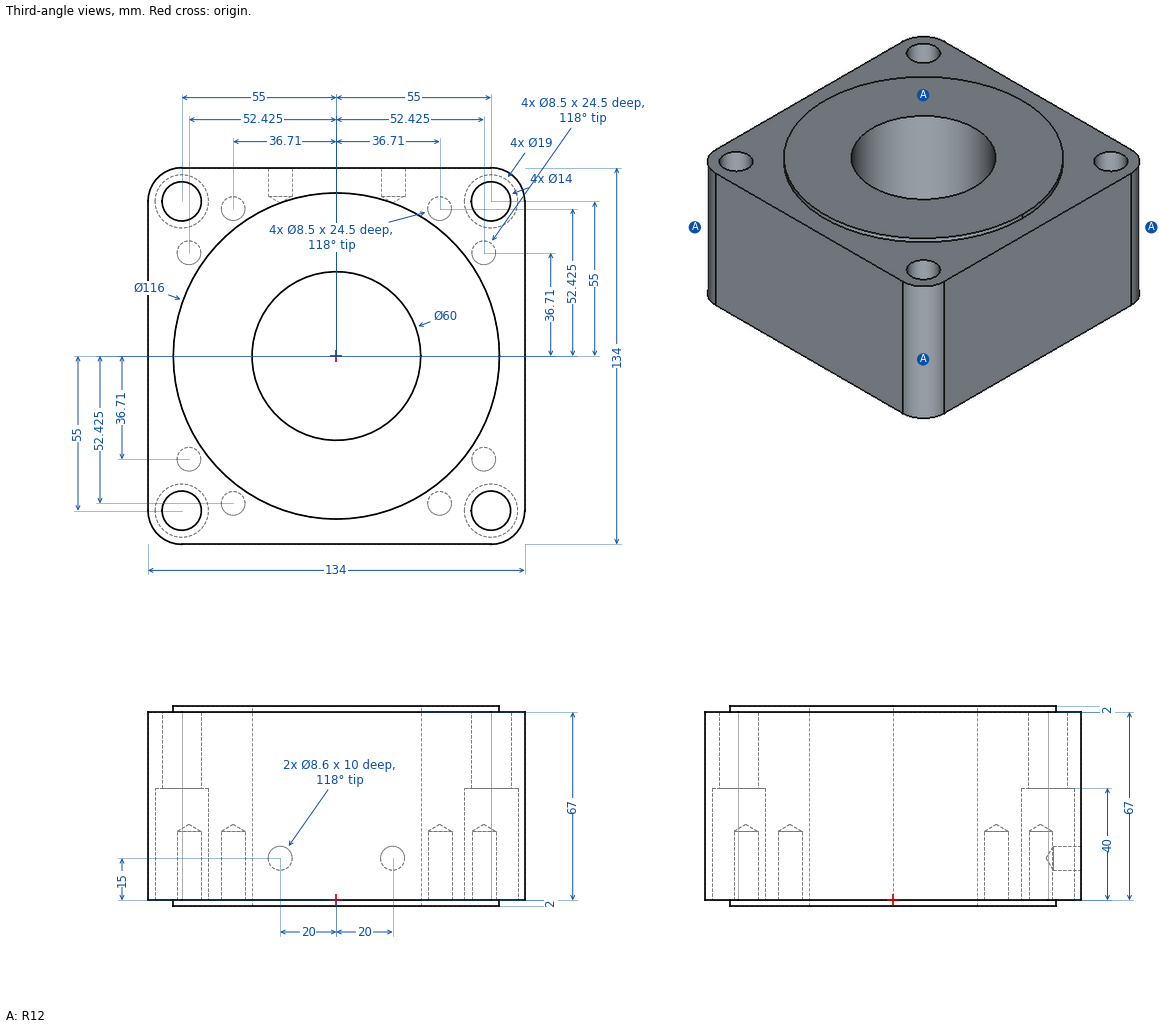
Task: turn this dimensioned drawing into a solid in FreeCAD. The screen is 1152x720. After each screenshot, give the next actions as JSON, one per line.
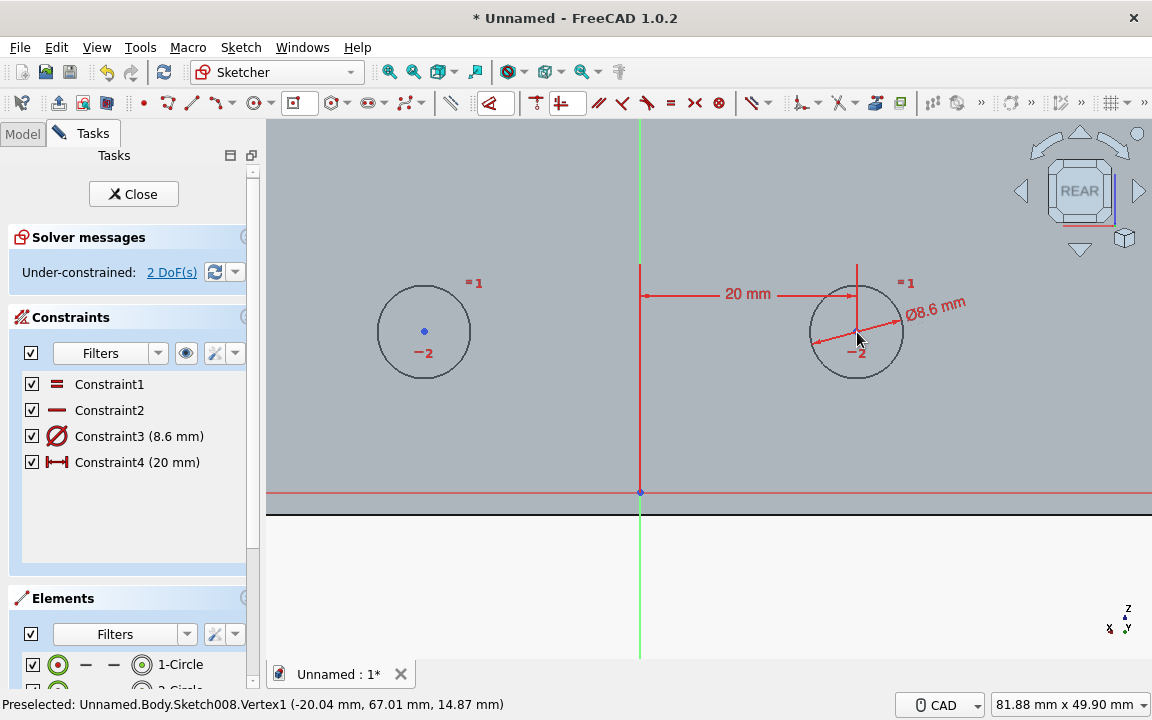
{"action": "left_click", "coordinate": [857, 332]}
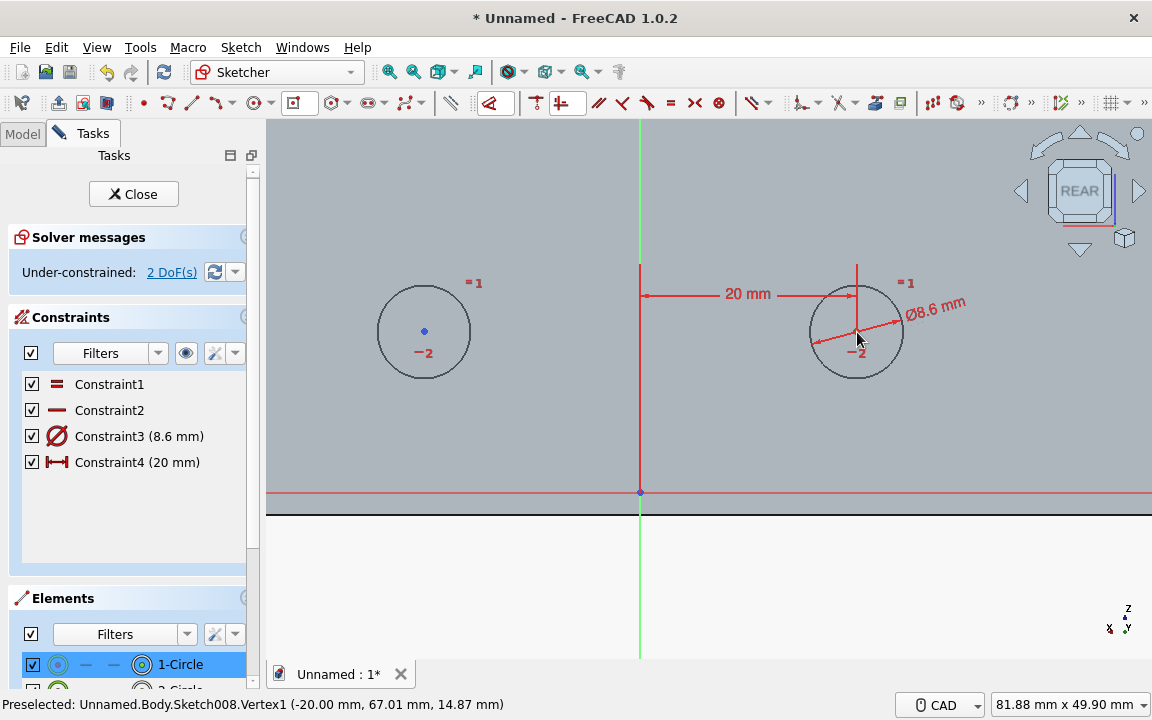
{"action": "key", "text": "i"}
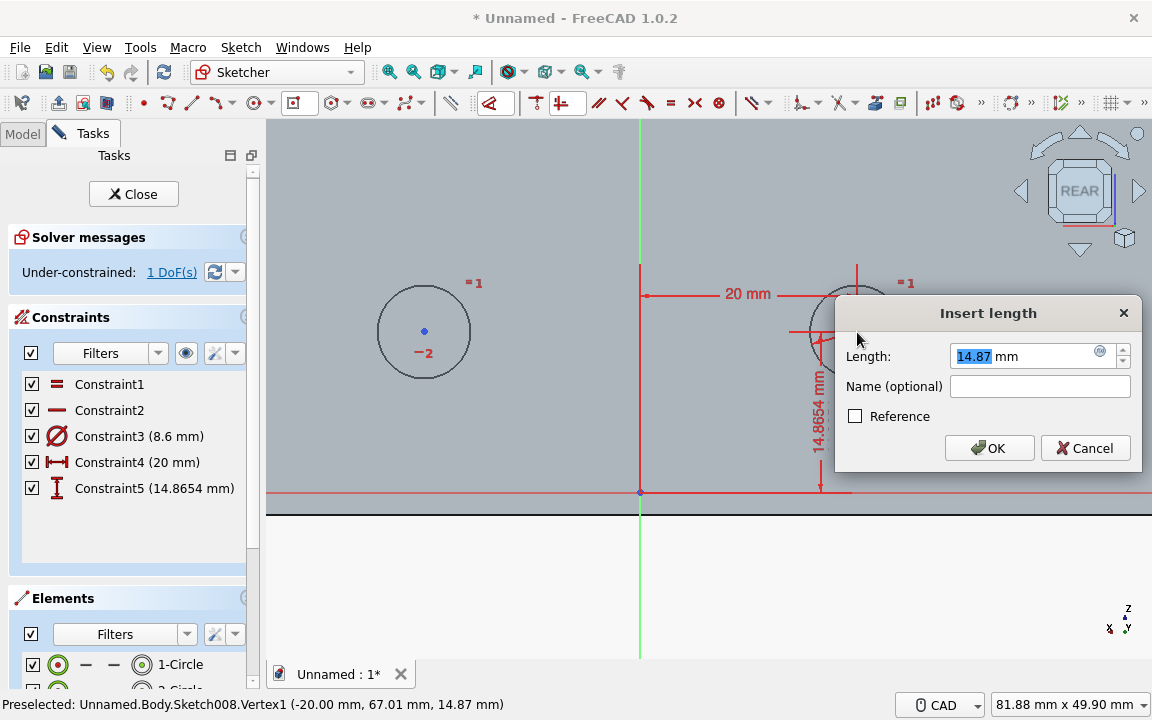
{"action": "type", "text": "15"}
{"action": "key", "text": "Return"}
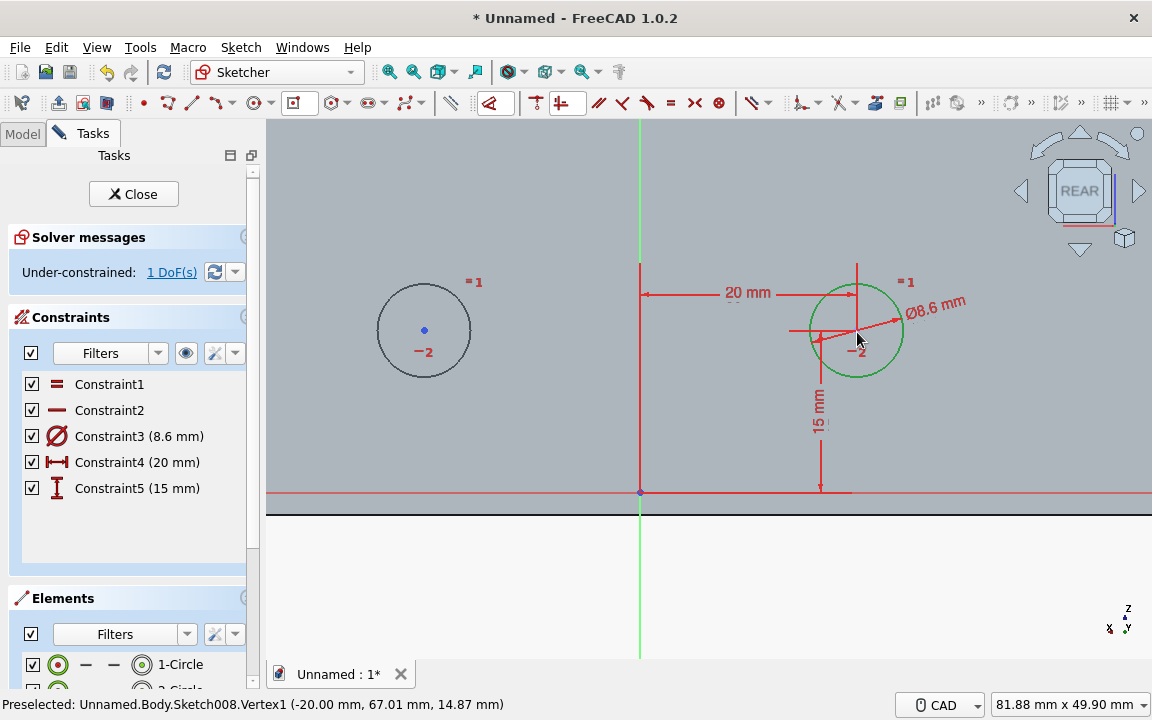
{"action": "left_click", "coordinate": [424, 331]}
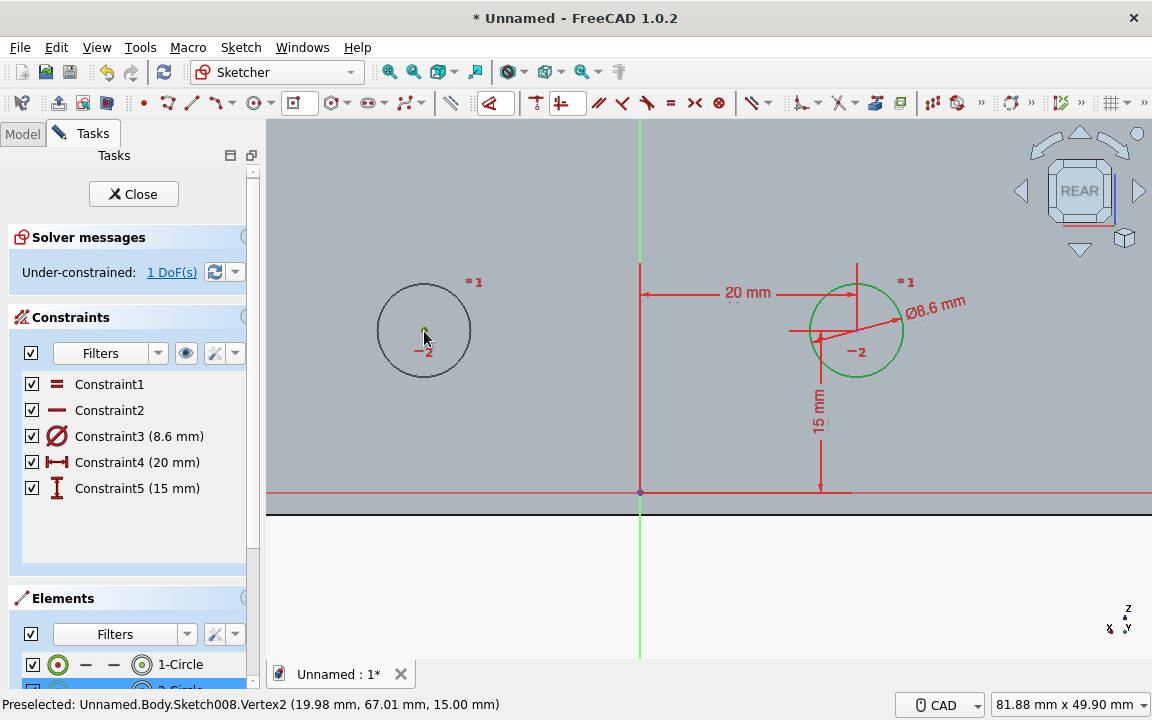
{"action": "left_click", "coordinate": [508, 104]}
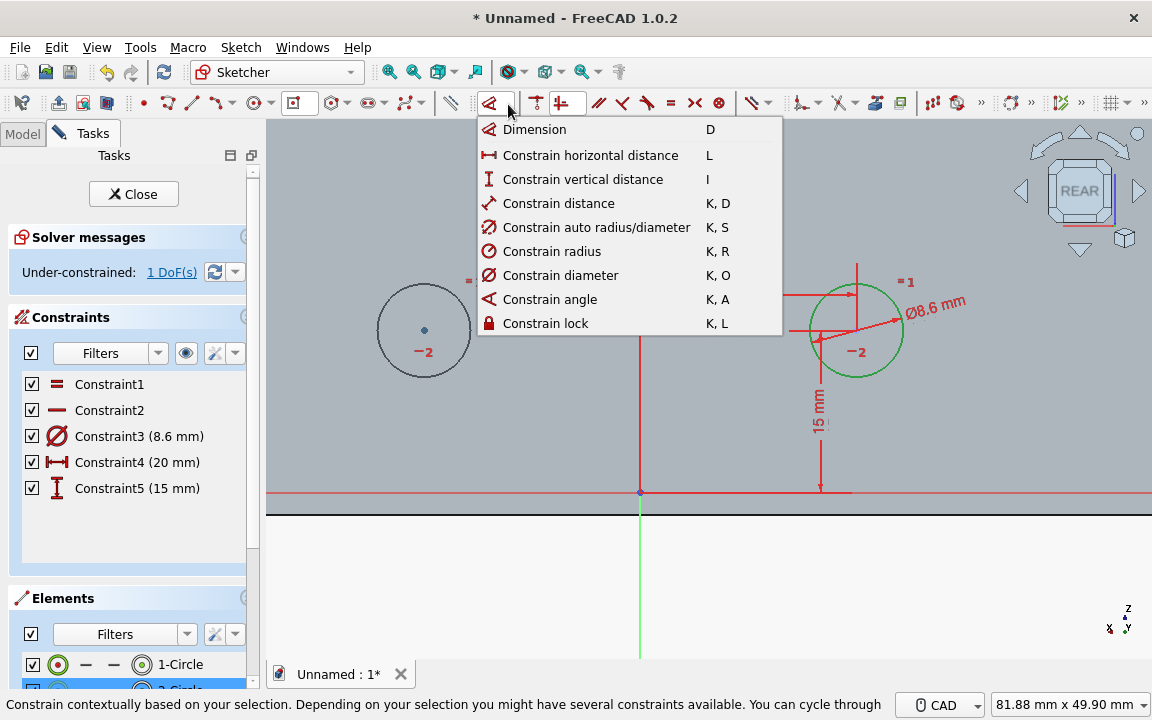
{"action": "left_click", "coordinate": [630, 155]}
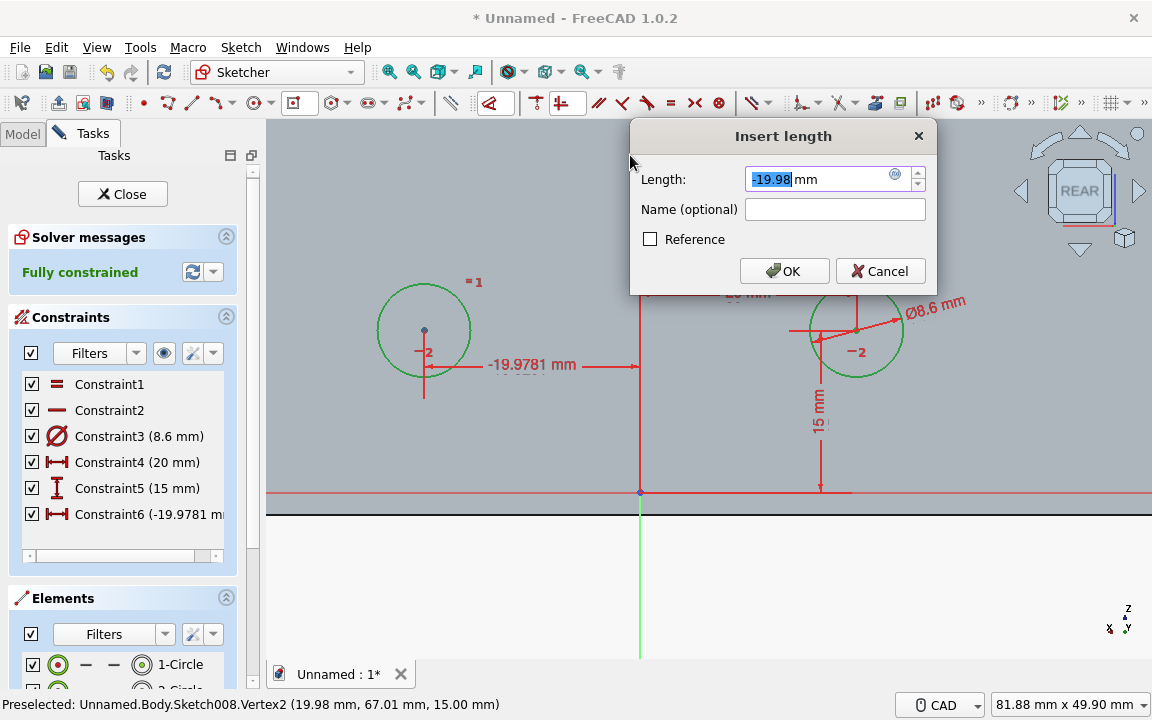
{"action": "type", "text": "-20"}
{"action": "key", "text": "Return"}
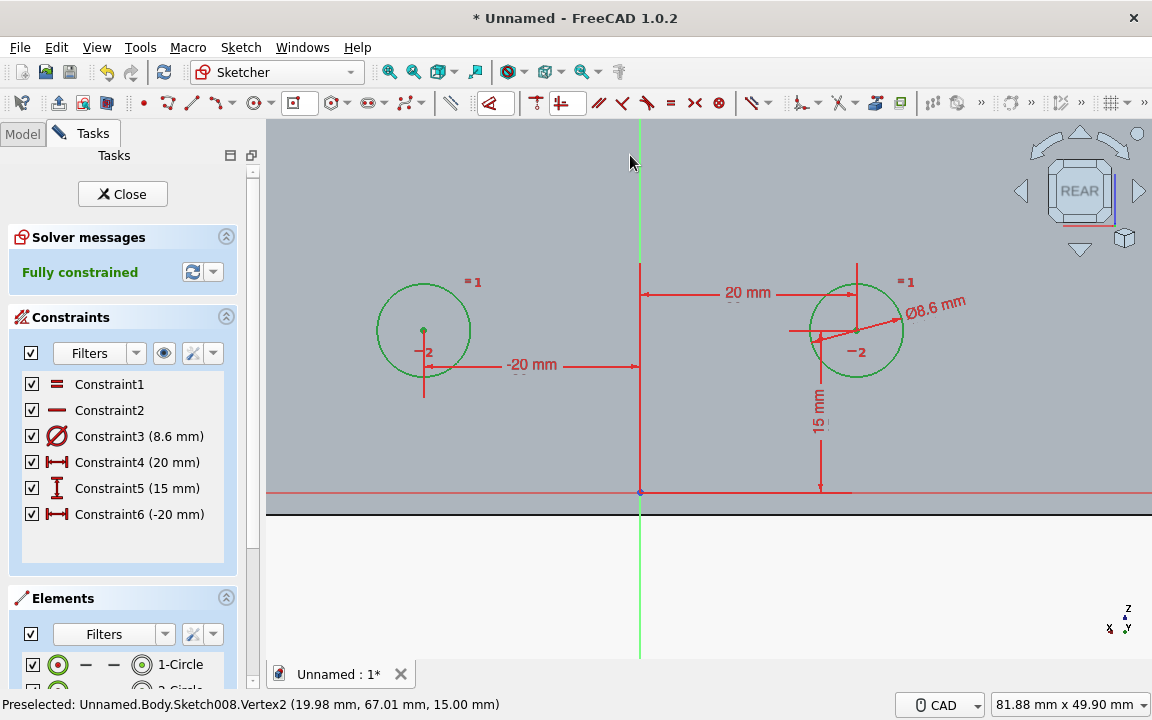
{"action": "left_click", "coordinate": [123, 194]}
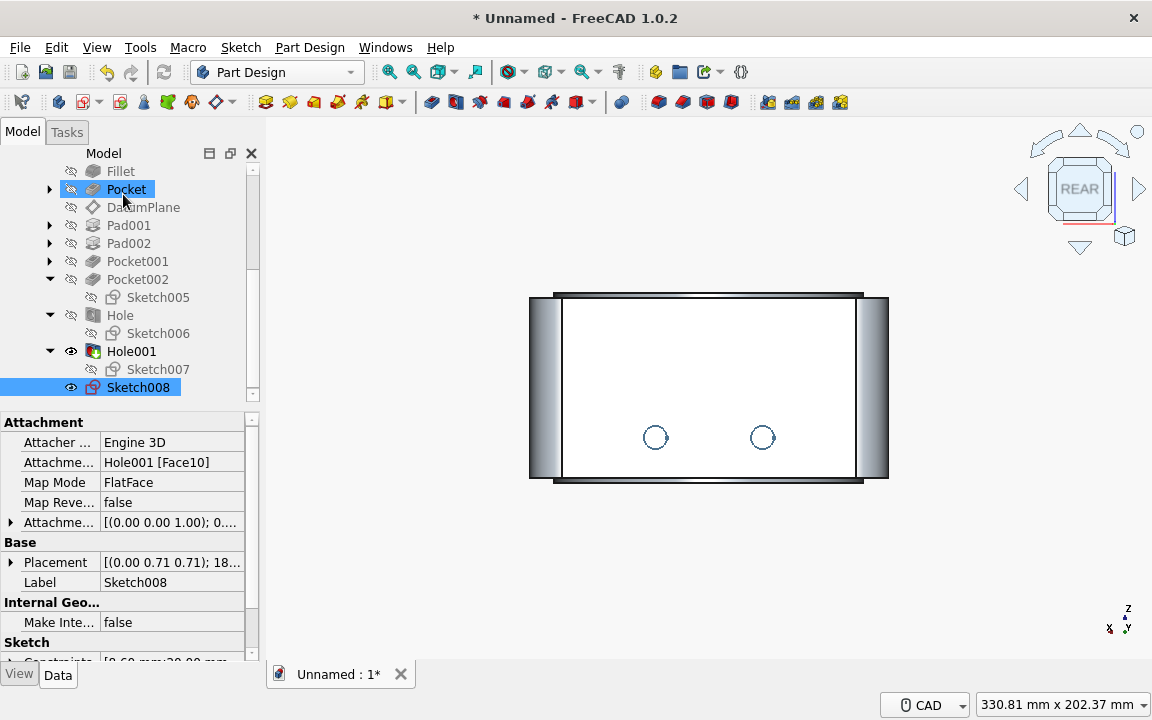
{"action": "left_click", "coordinate": [456, 102]}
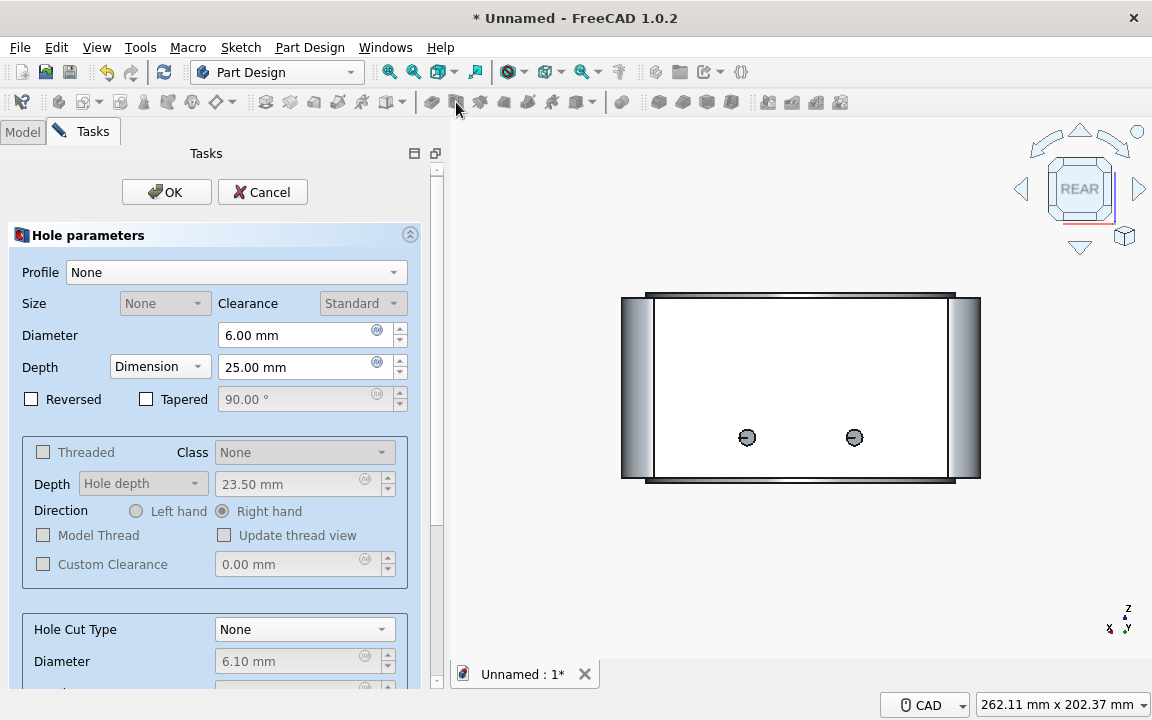
{"action": "triple_click", "coordinate": [305, 335]}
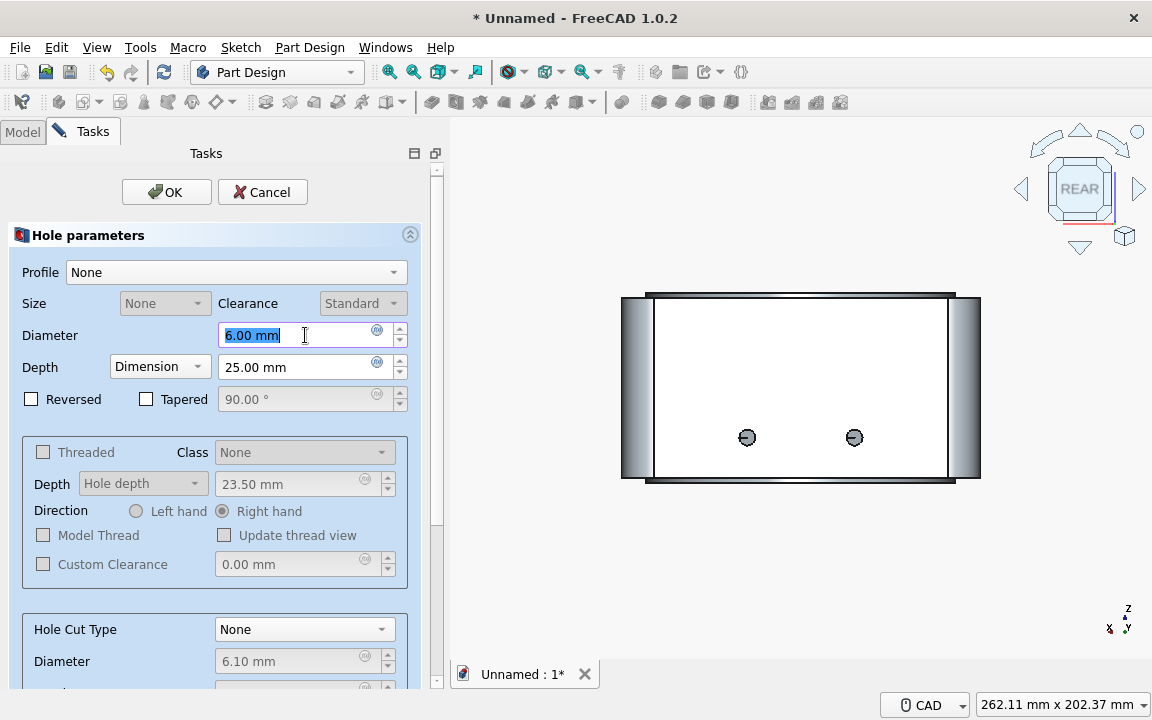
{"action": "type", "text": "8.6"}
{"action": "key", "text": "Tab"}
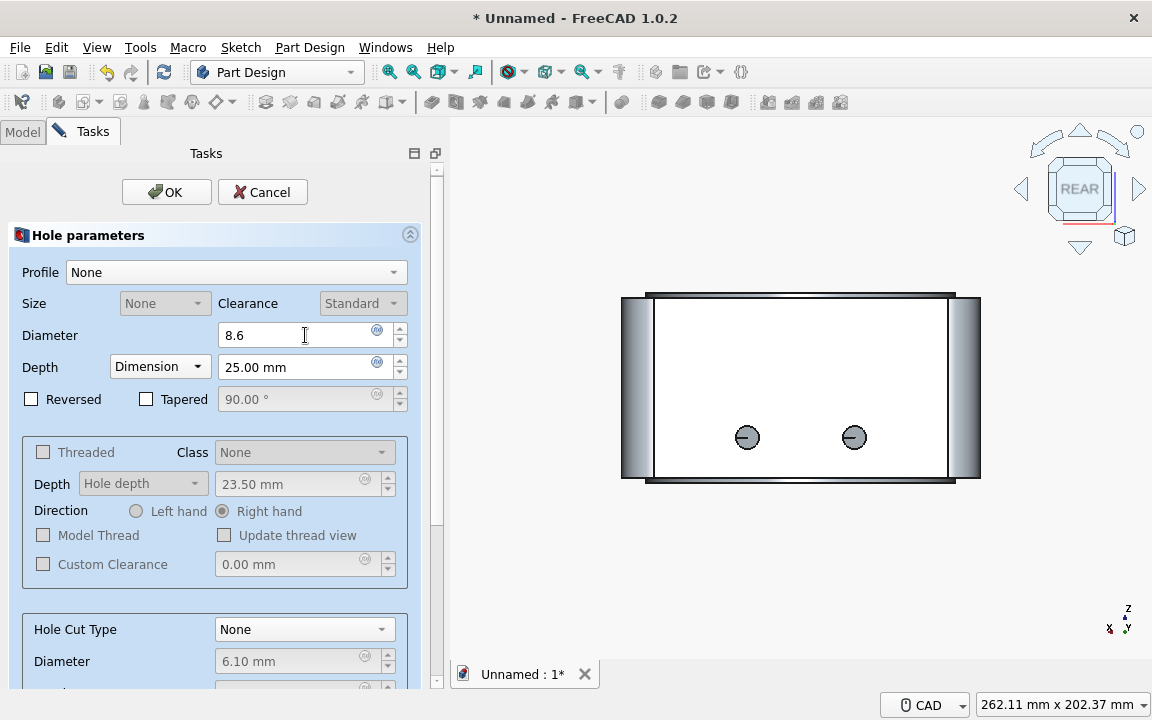
{"action": "triple_click", "coordinate": [305, 367]}